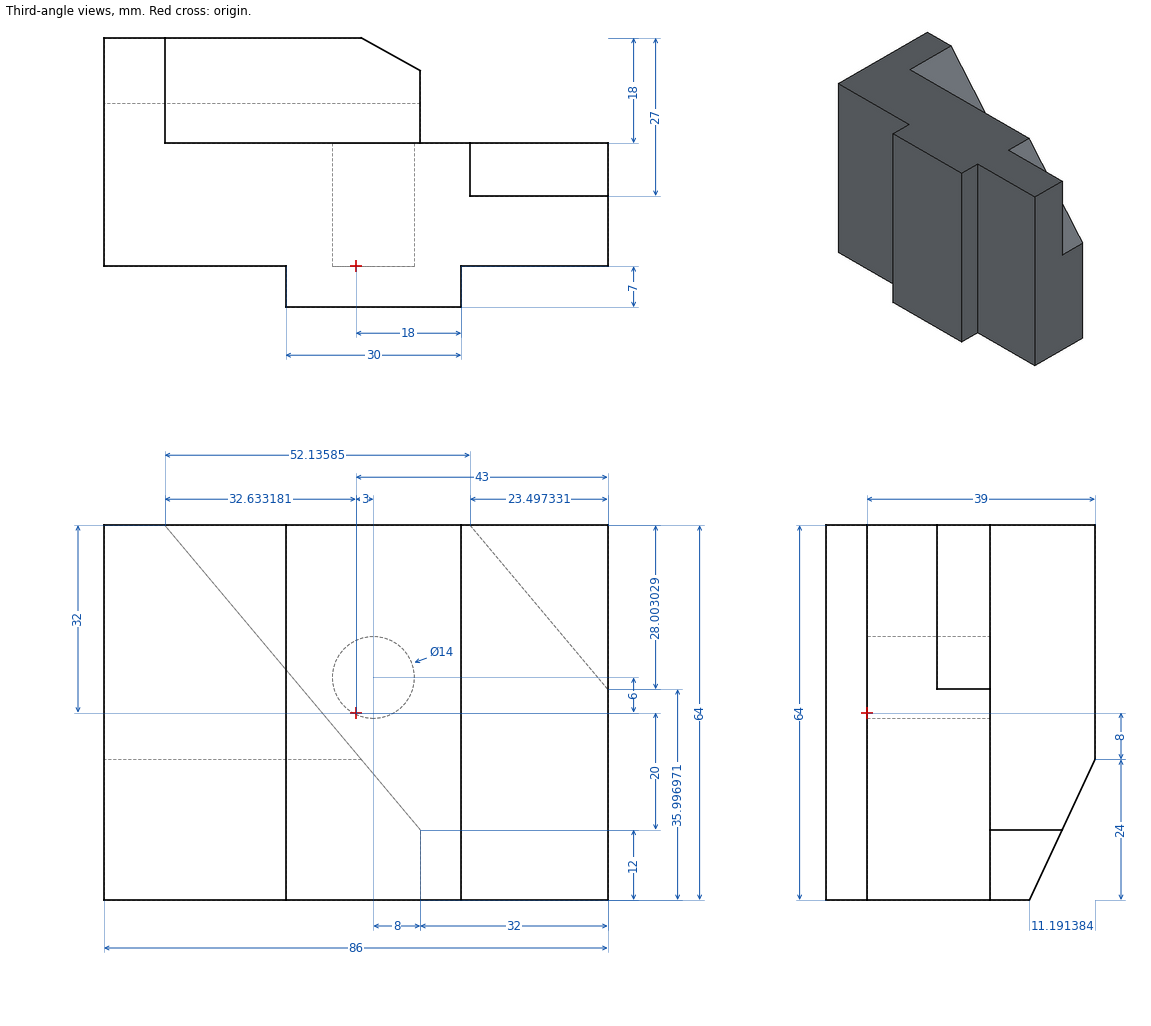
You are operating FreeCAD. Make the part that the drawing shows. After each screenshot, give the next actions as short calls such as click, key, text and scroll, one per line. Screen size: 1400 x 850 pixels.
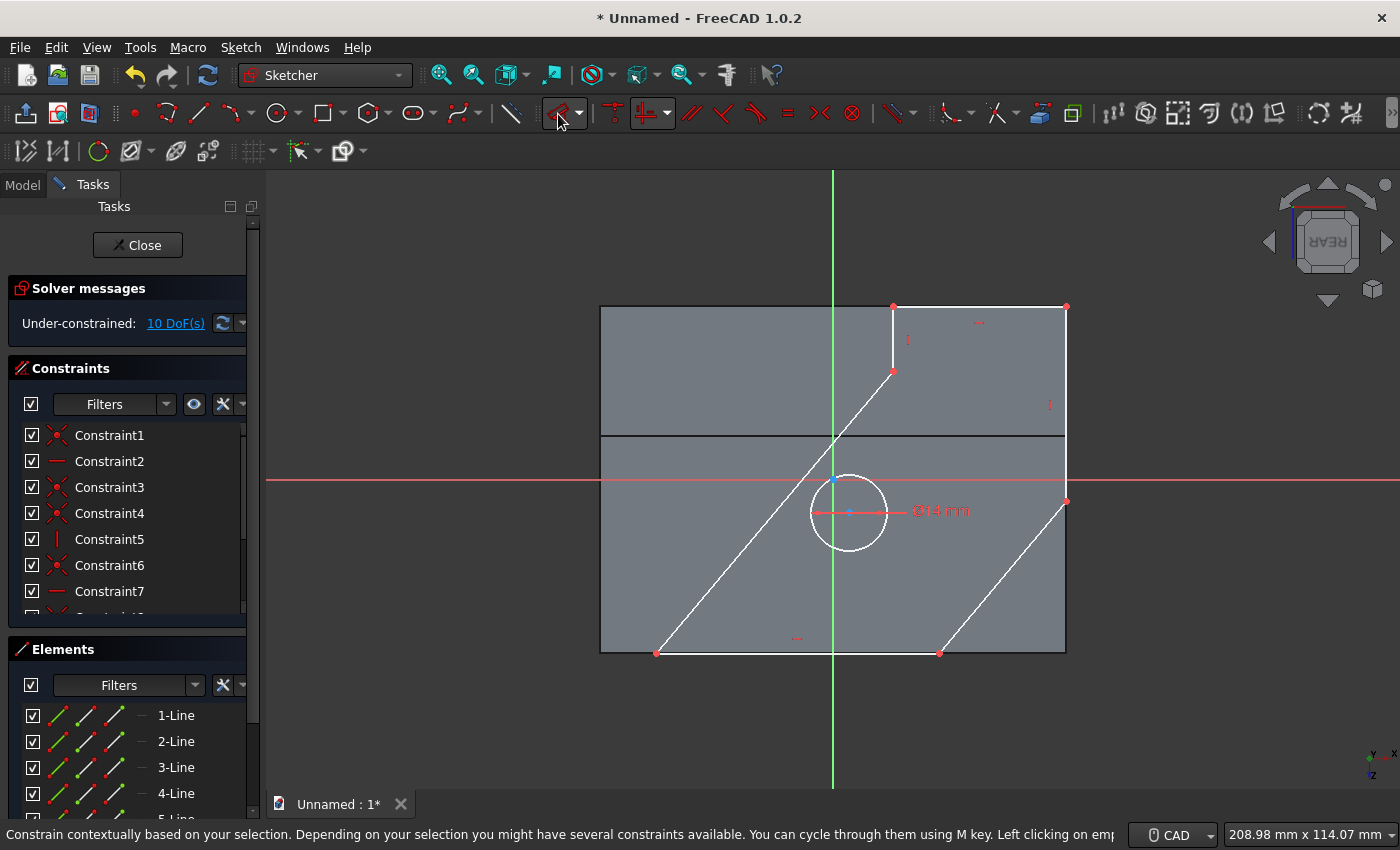
scroll(849, 513, up, 5)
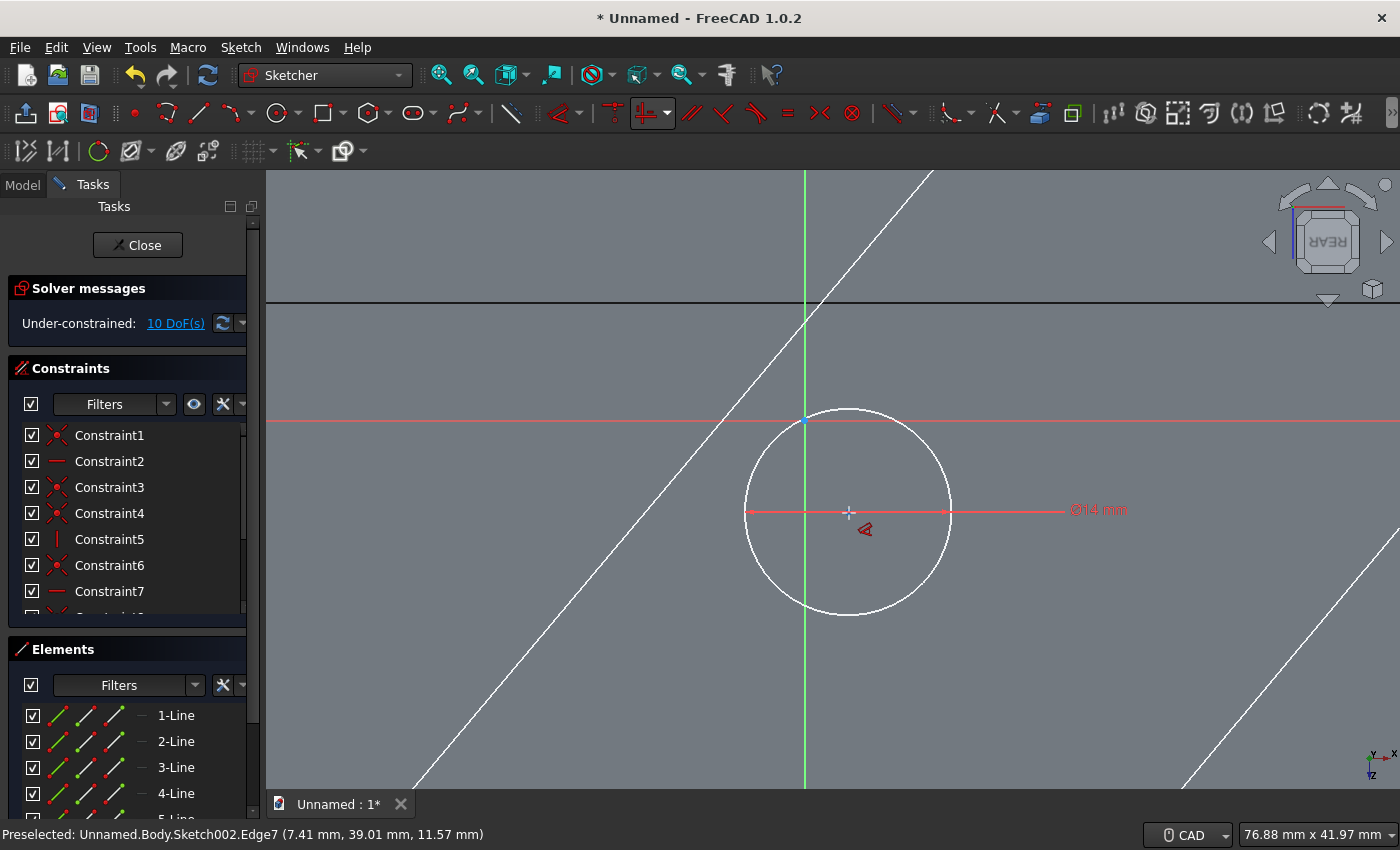
click(848, 512)
click(826, 546)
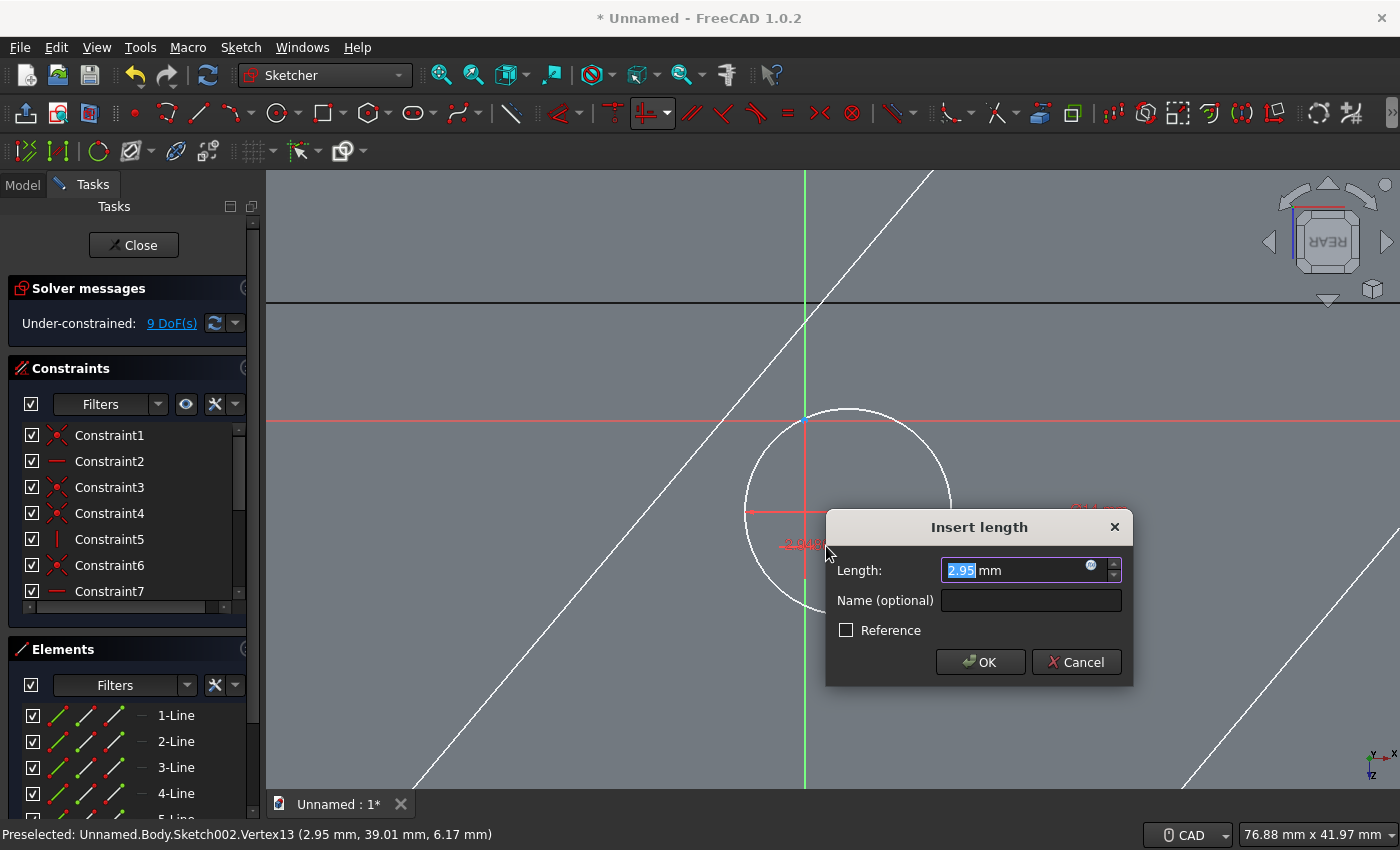
text(3)
key(Return)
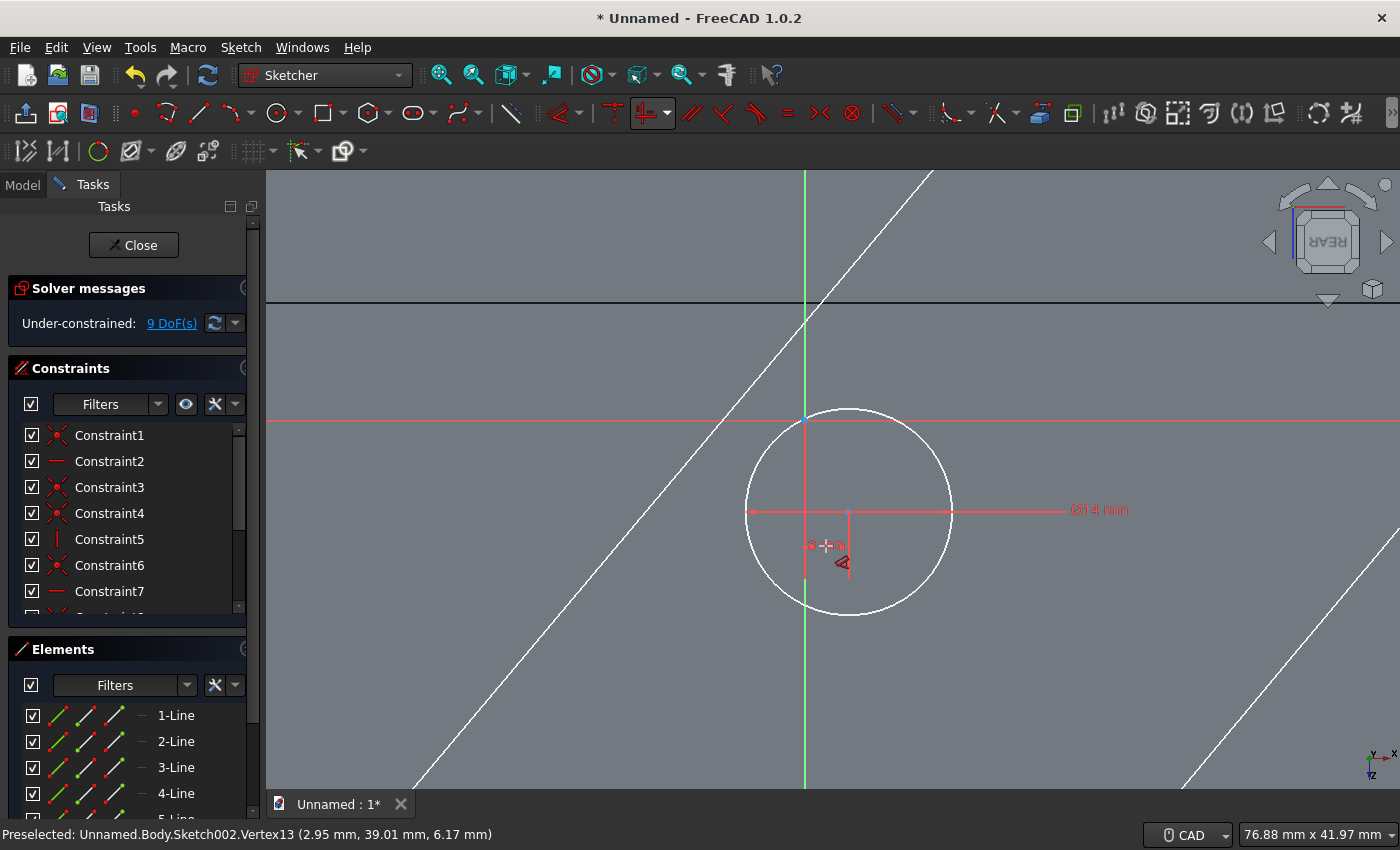
click(849, 512)
click(771, 487)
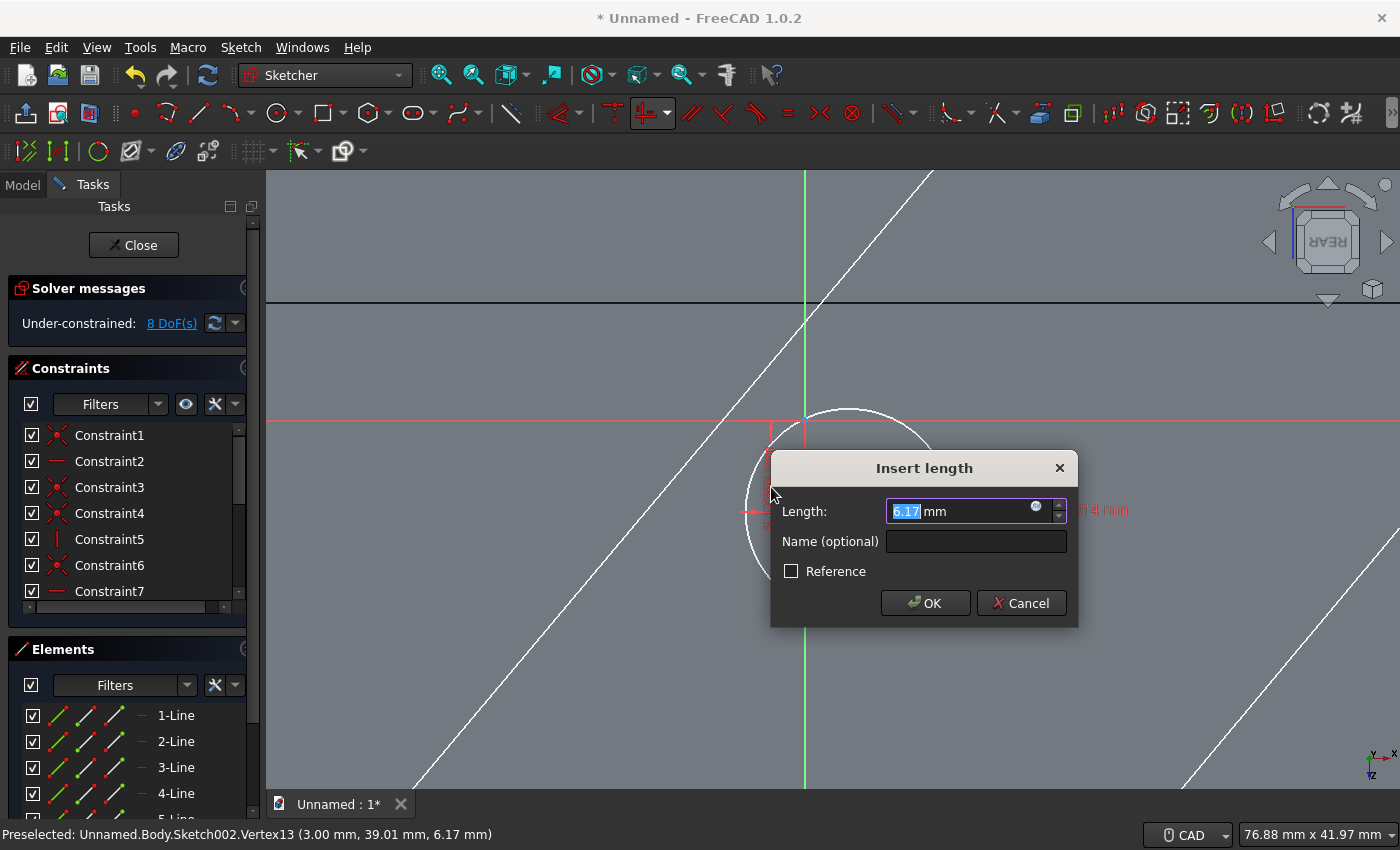
text(6)
key(Return)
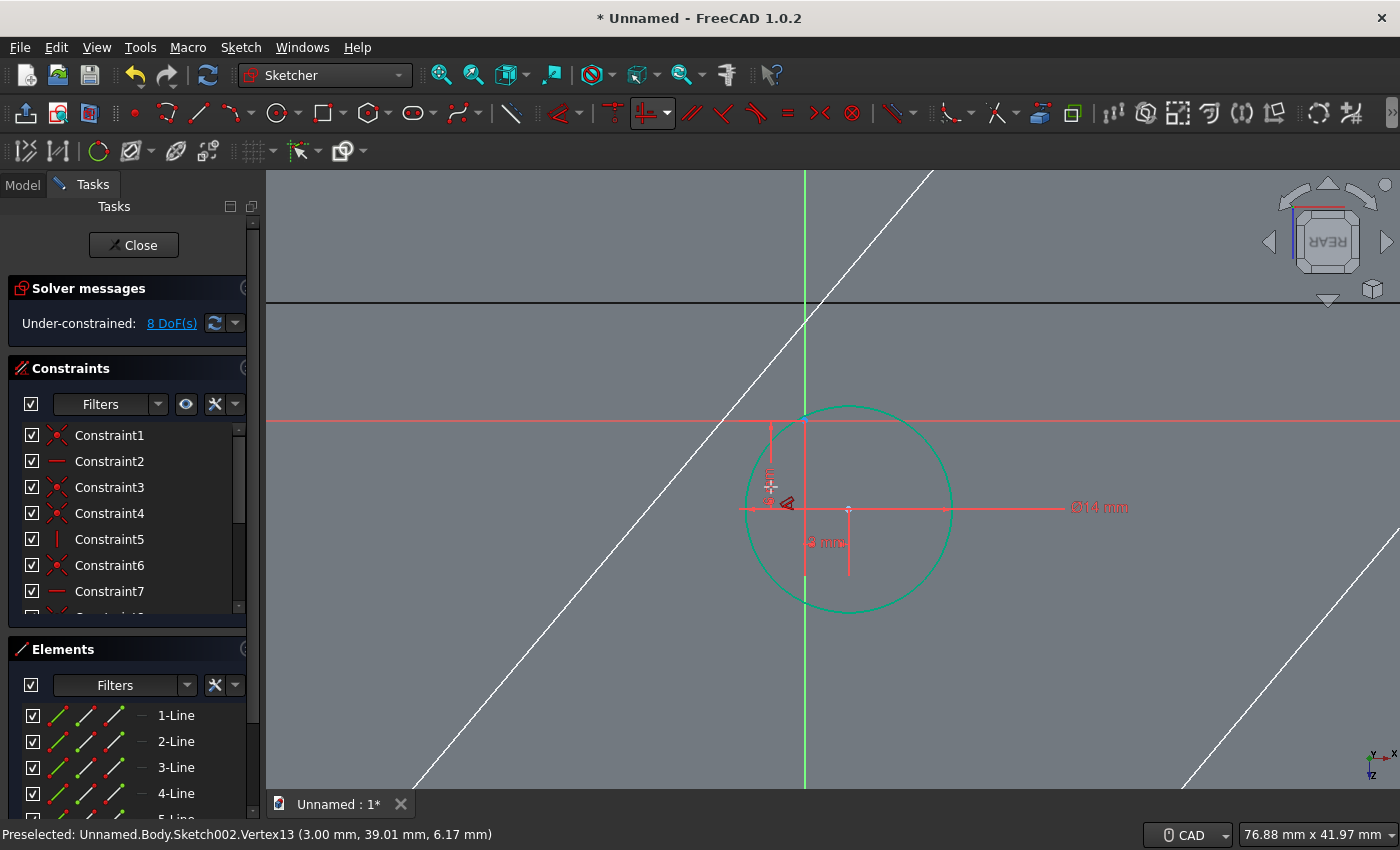
scroll(669, 527, down, 4)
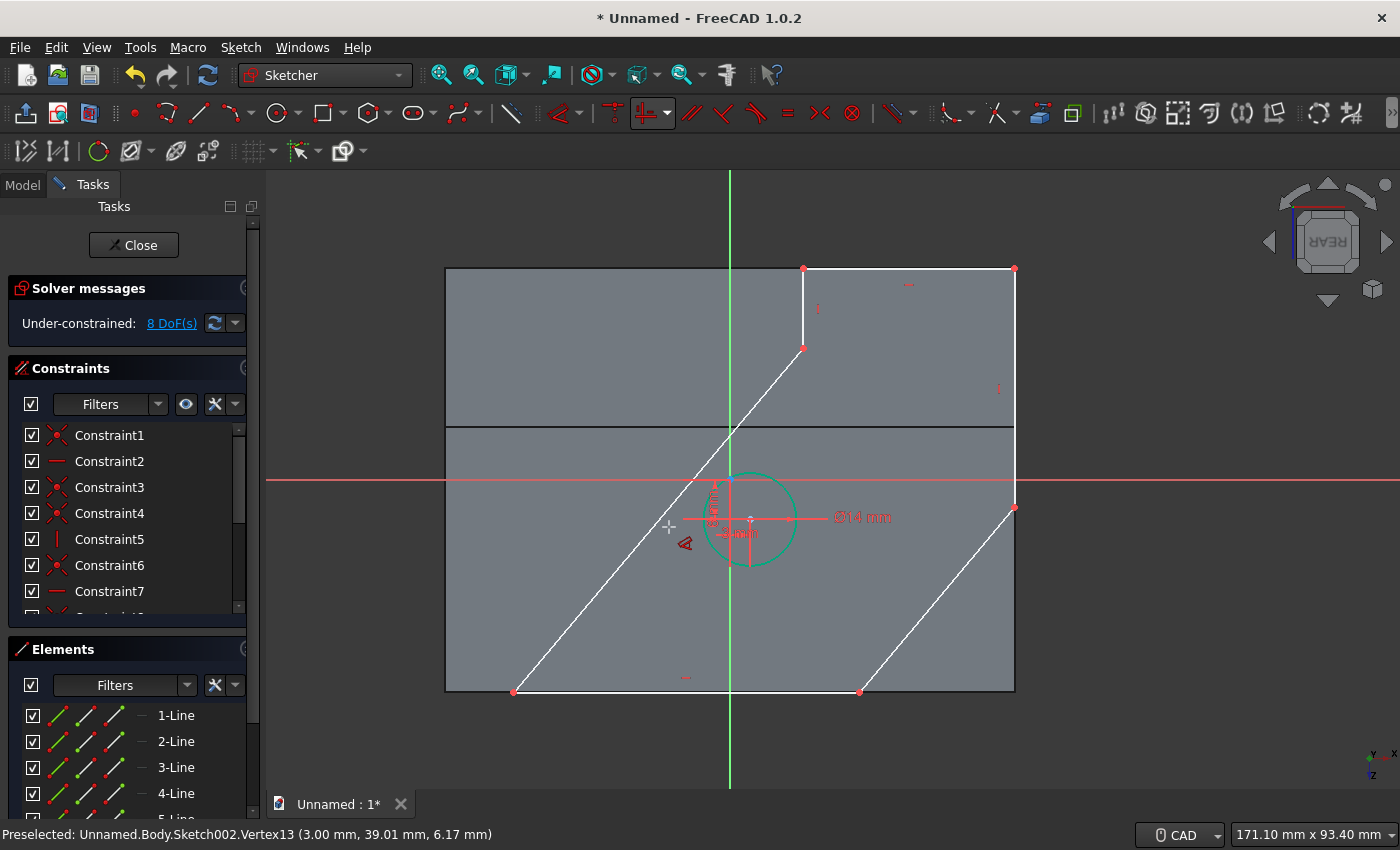
click(951, 269)
click(909, 235)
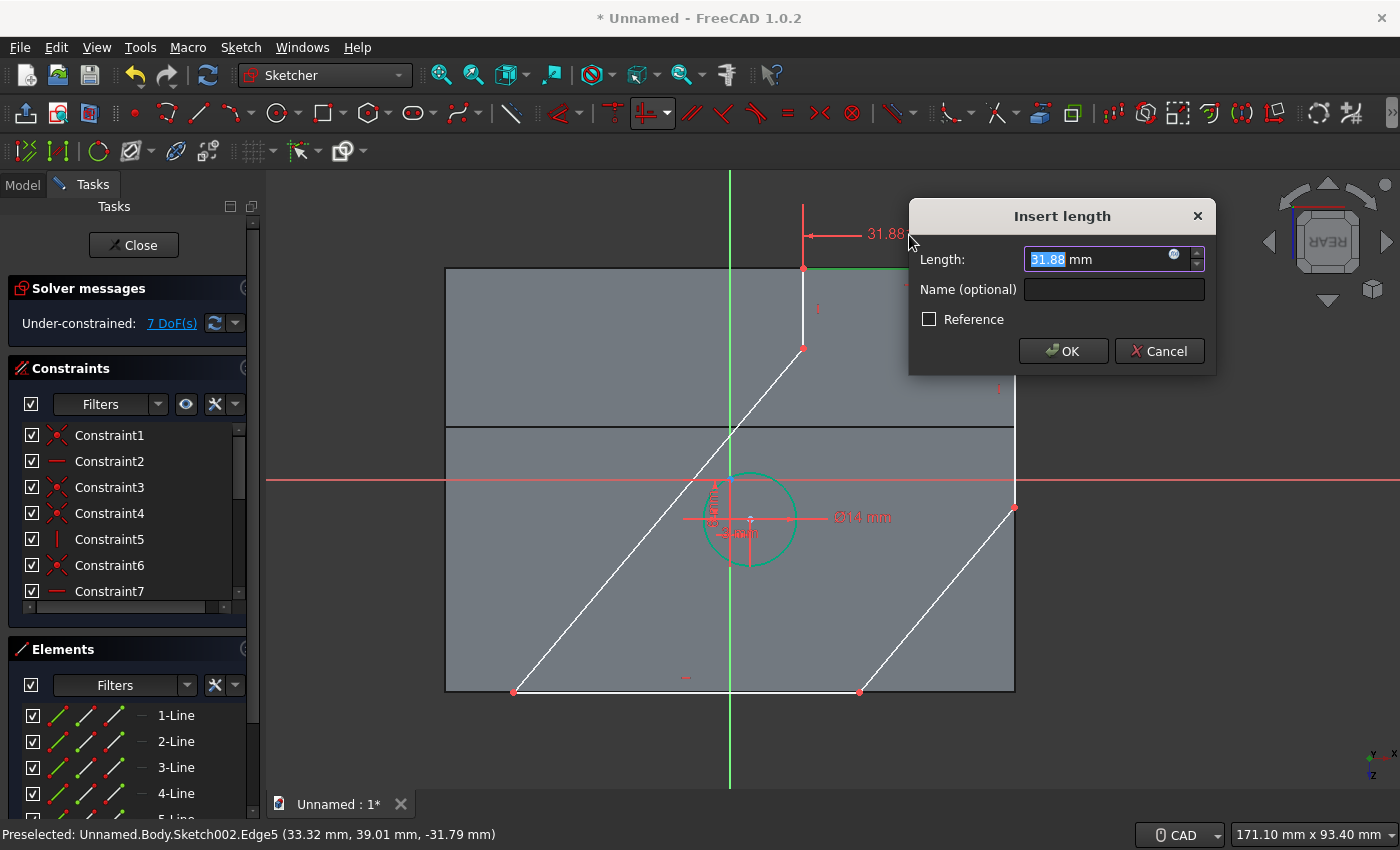
text(32)
key(Return)